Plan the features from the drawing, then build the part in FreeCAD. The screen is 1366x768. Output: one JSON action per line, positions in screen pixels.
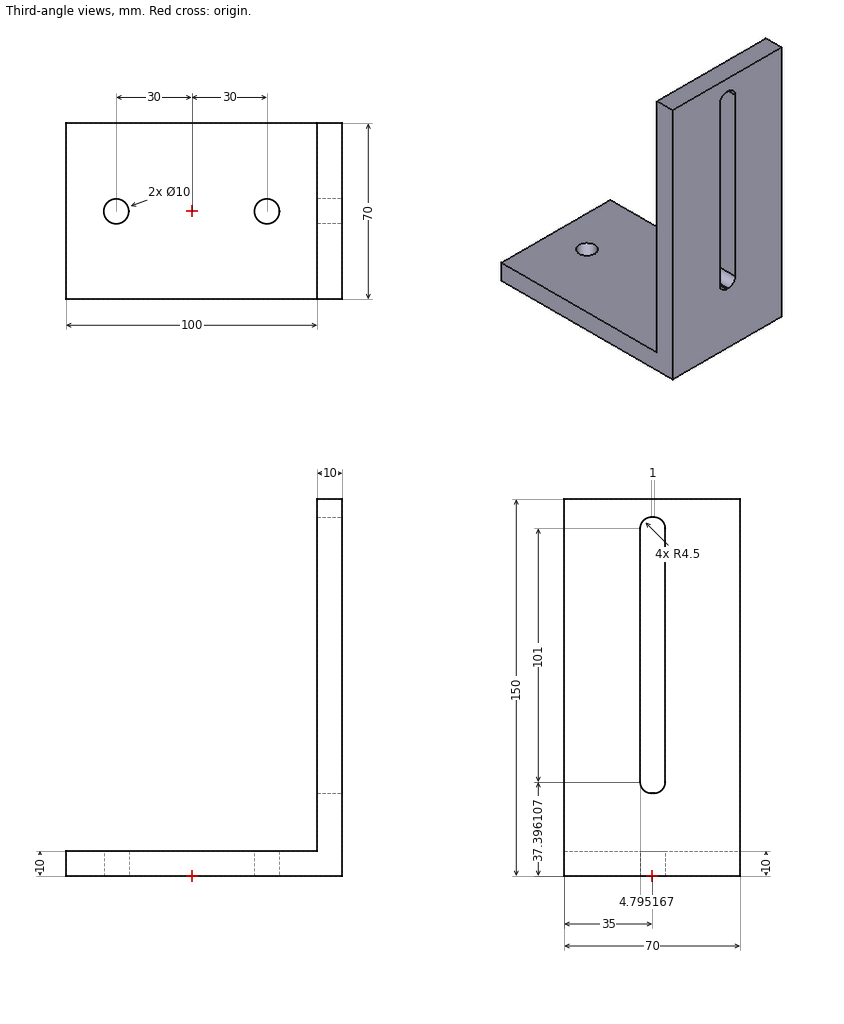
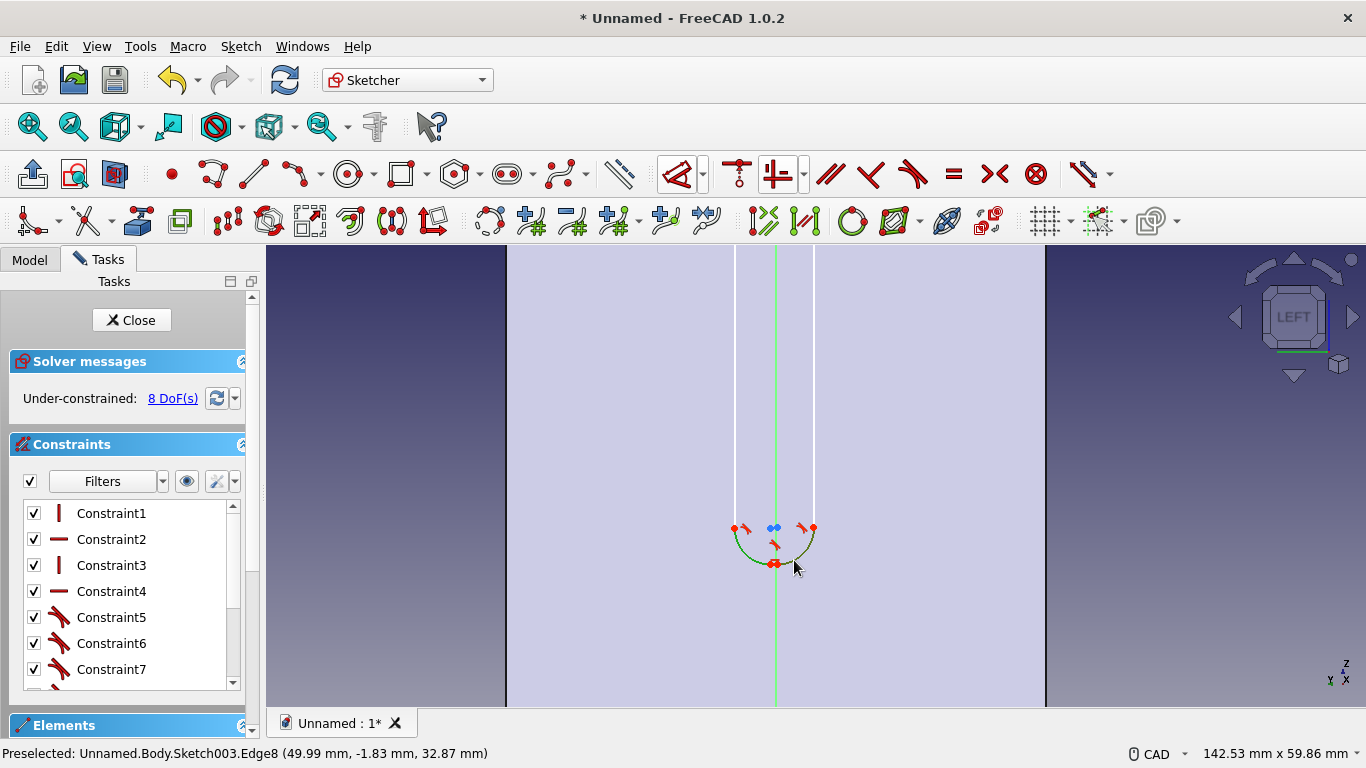
{"action": "left_click", "coordinate": [954, 174]}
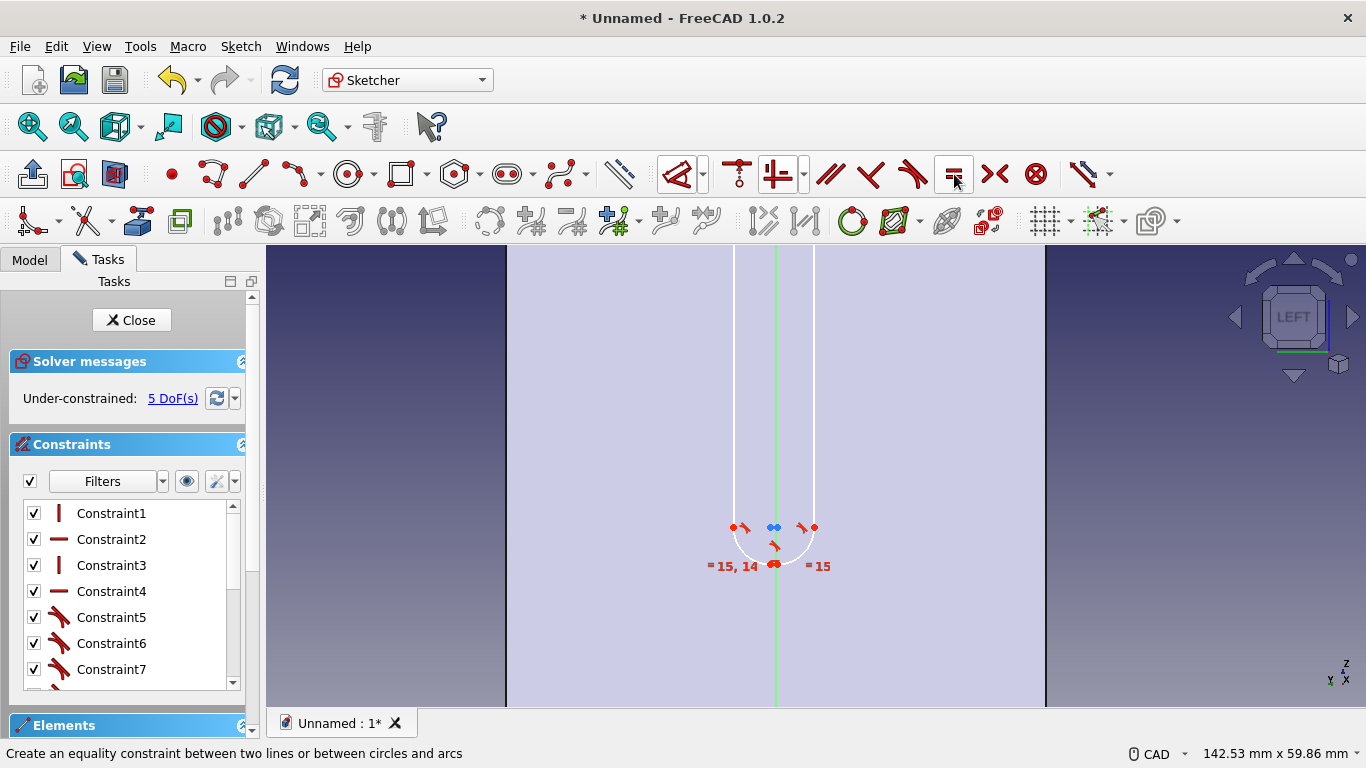
{"action": "scroll", "coordinate": [739, 545], "scroll_direction": "down", "scroll_amount": 7}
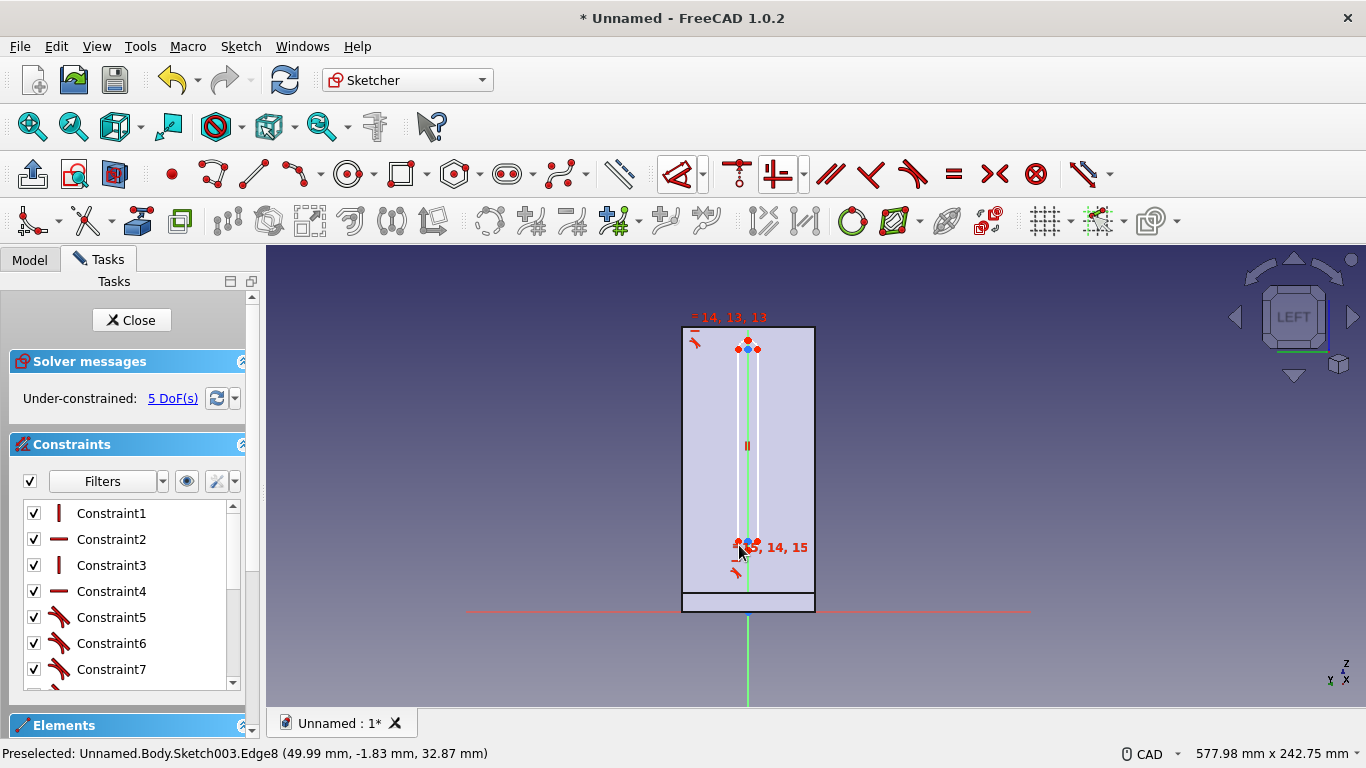
{"action": "scroll", "coordinate": [757, 345], "scroll_direction": "up", "scroll_amount": 8}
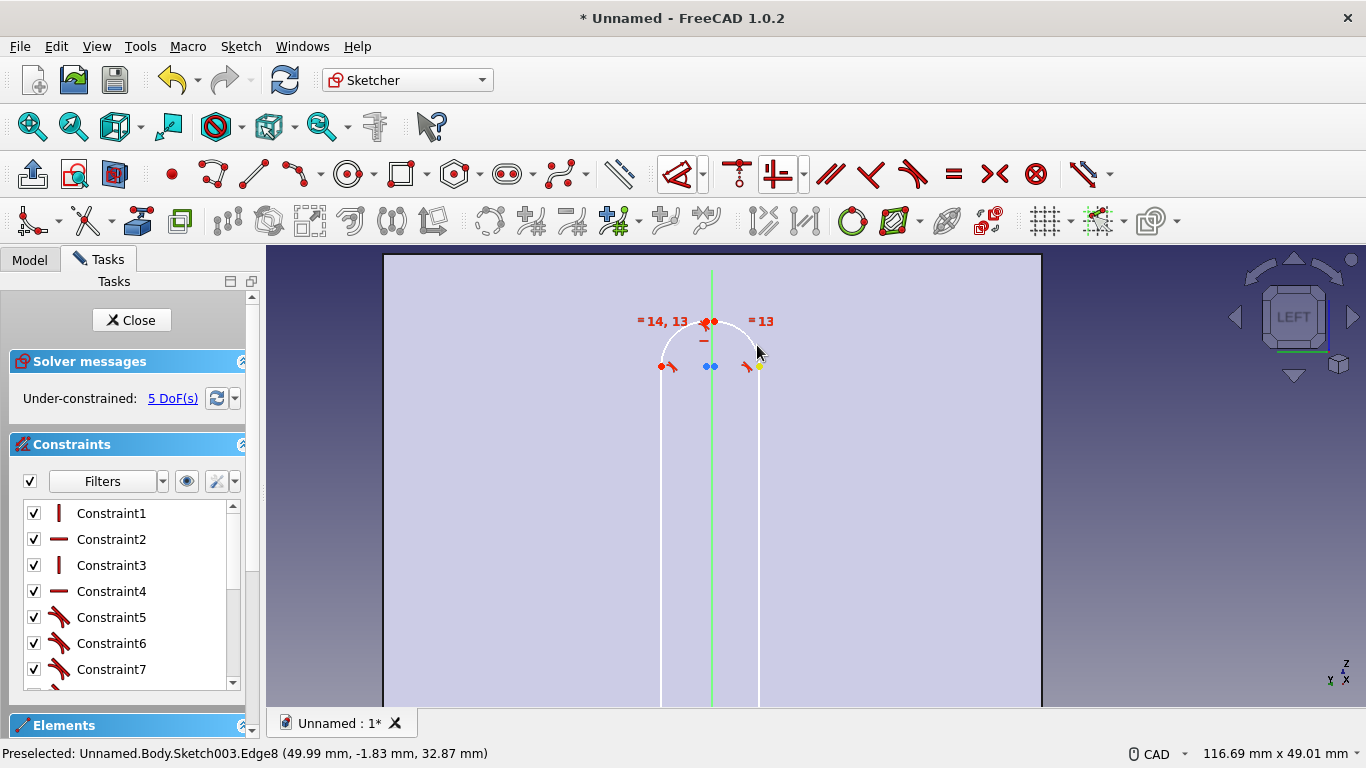
{"action": "left_click", "coordinate": [754, 346]}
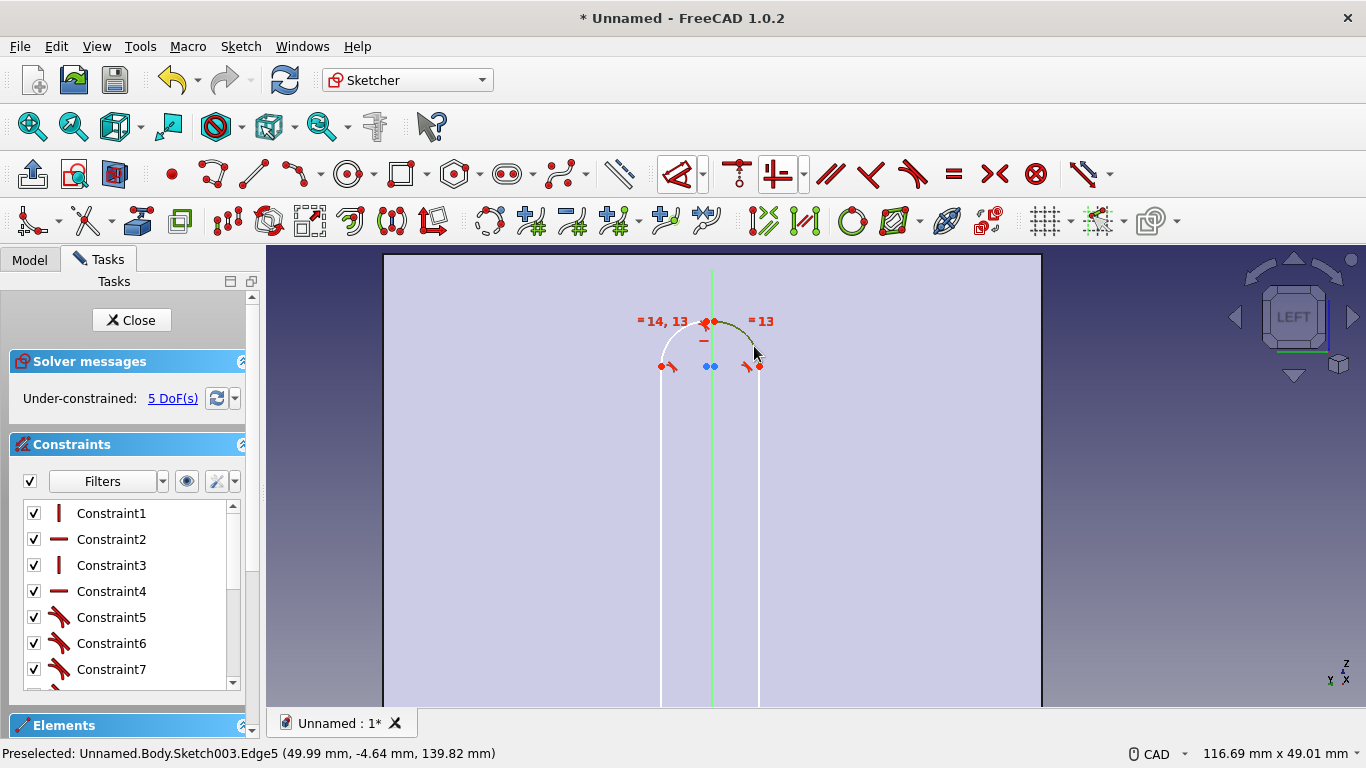
{"action": "key", "text": "k r"}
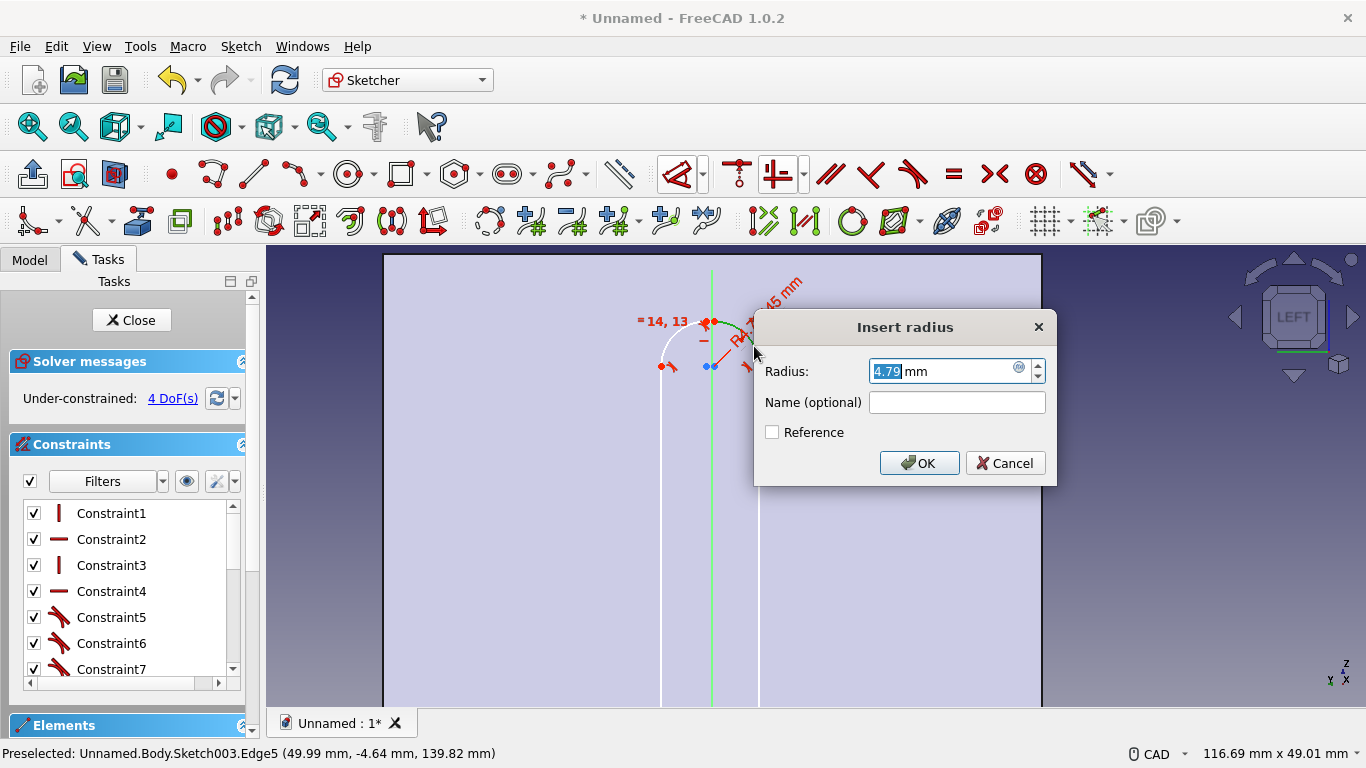
{"action": "type", "text": "4.5"}
{"action": "key", "text": "Return"}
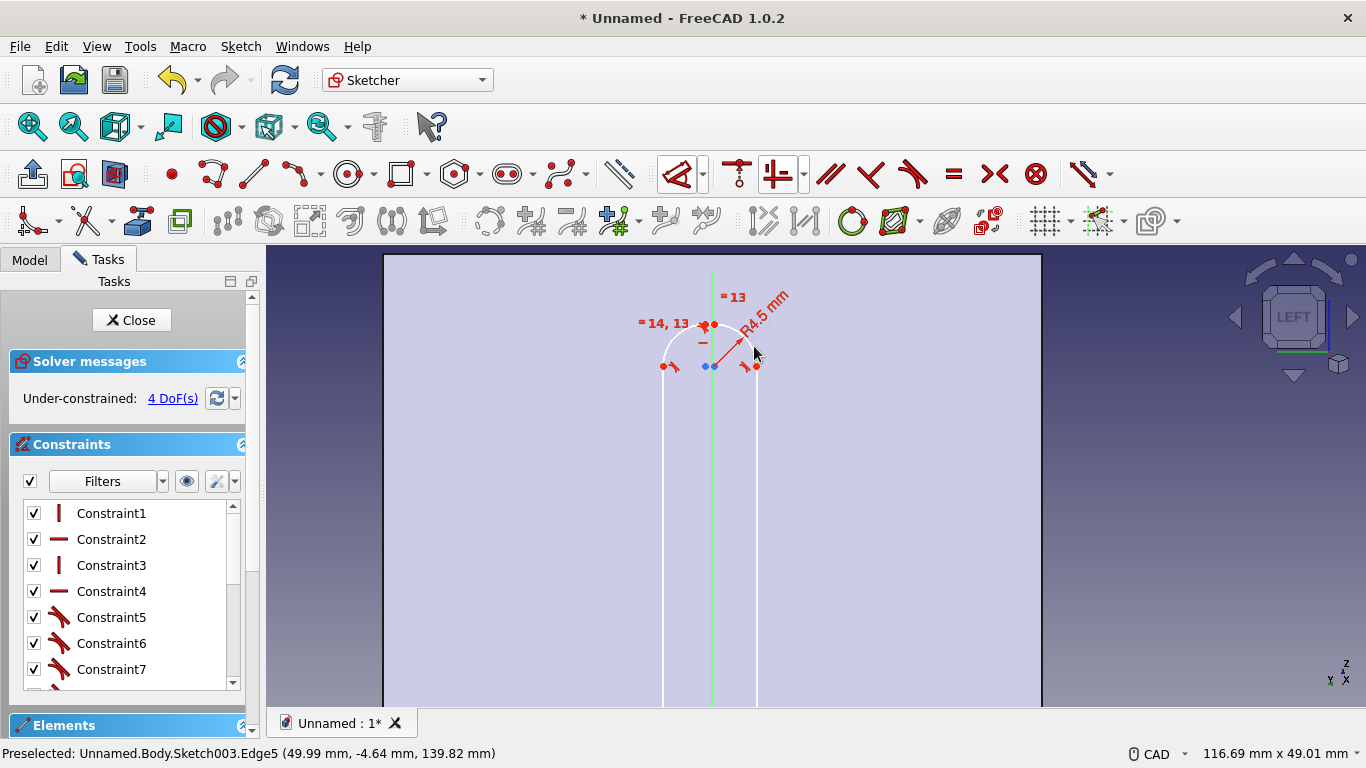
{"action": "scroll", "coordinate": [710, 324], "scroll_direction": "up", "scroll_amount": 8}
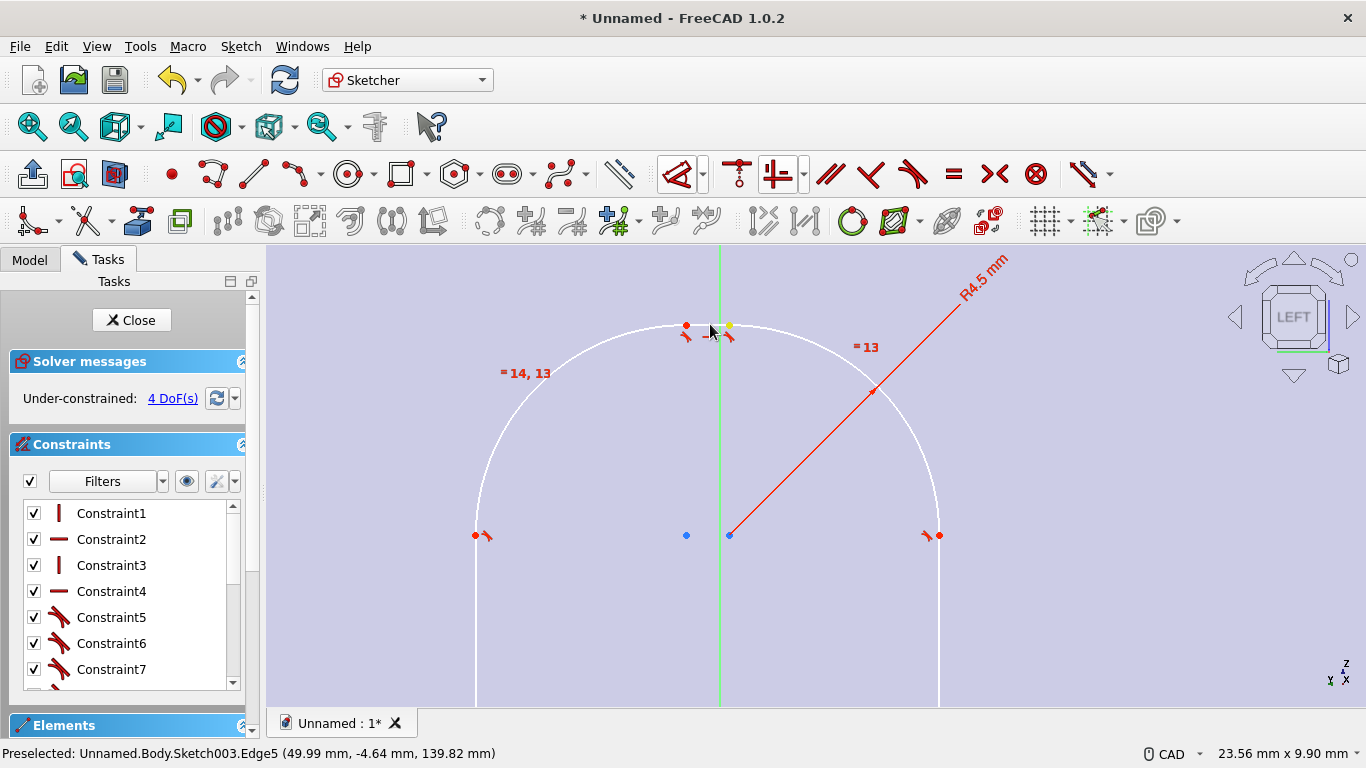
{"action": "left_click", "coordinate": [708, 325]}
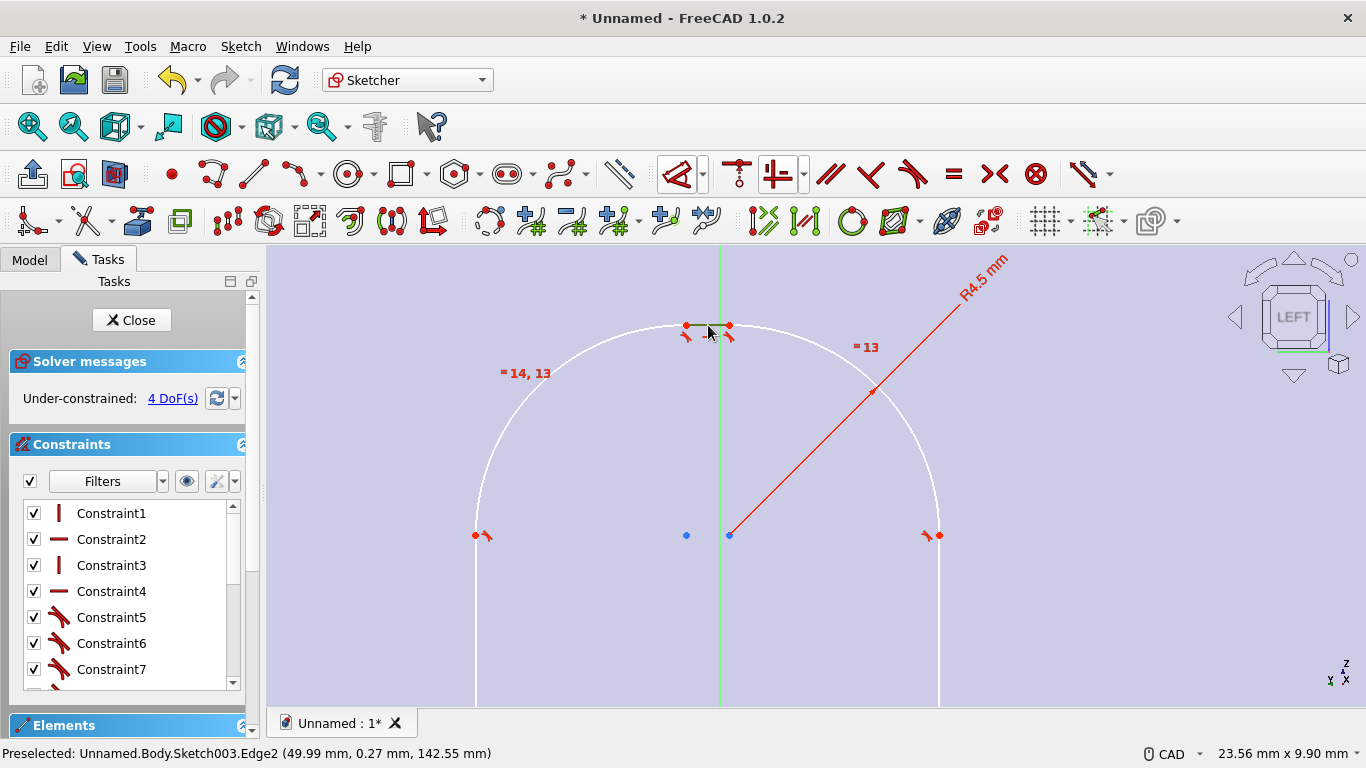
{"action": "left_click", "coordinate": [702, 174]}